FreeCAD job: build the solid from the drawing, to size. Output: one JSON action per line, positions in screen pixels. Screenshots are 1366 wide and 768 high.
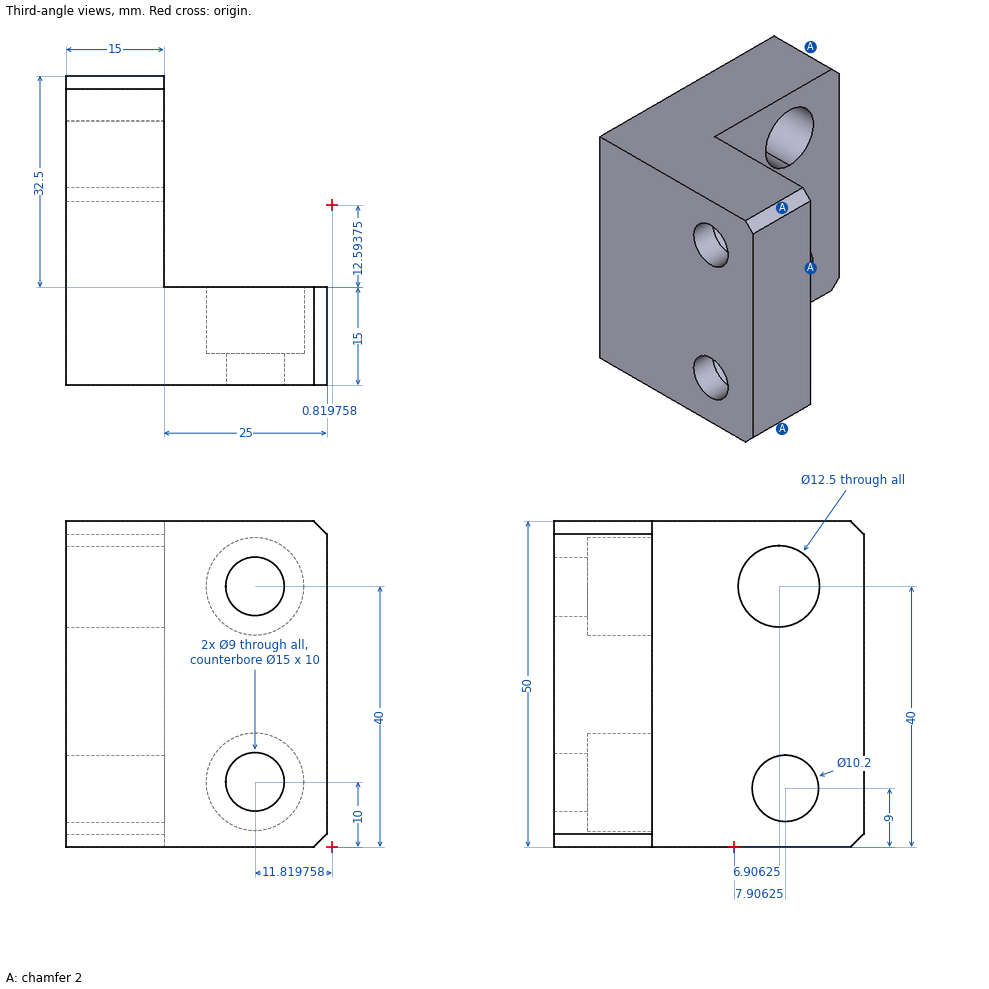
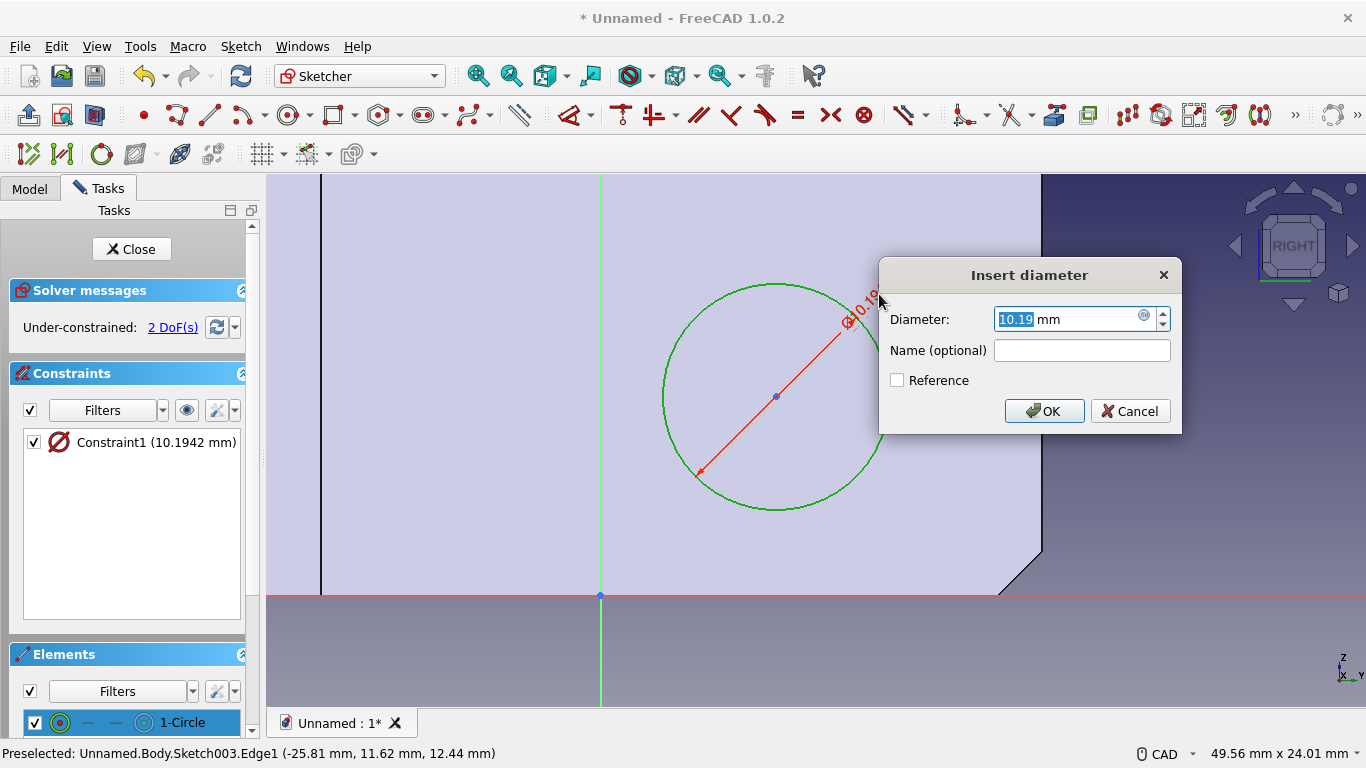
{"action": "type", "text": "10.2"}
{"action": "key", "text": "Return"}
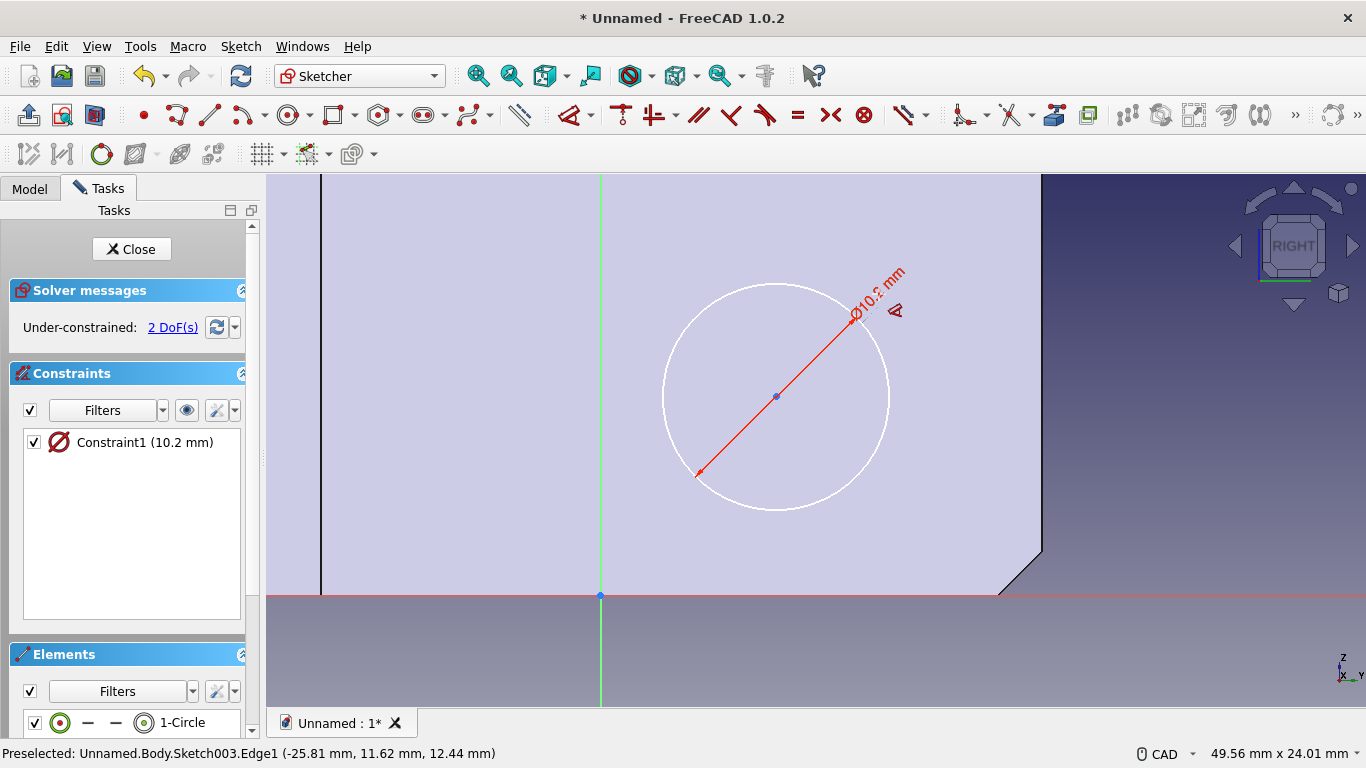
{"action": "left_click", "coordinate": [776, 397]}
{"action": "left_click", "coordinate": [567, 496]}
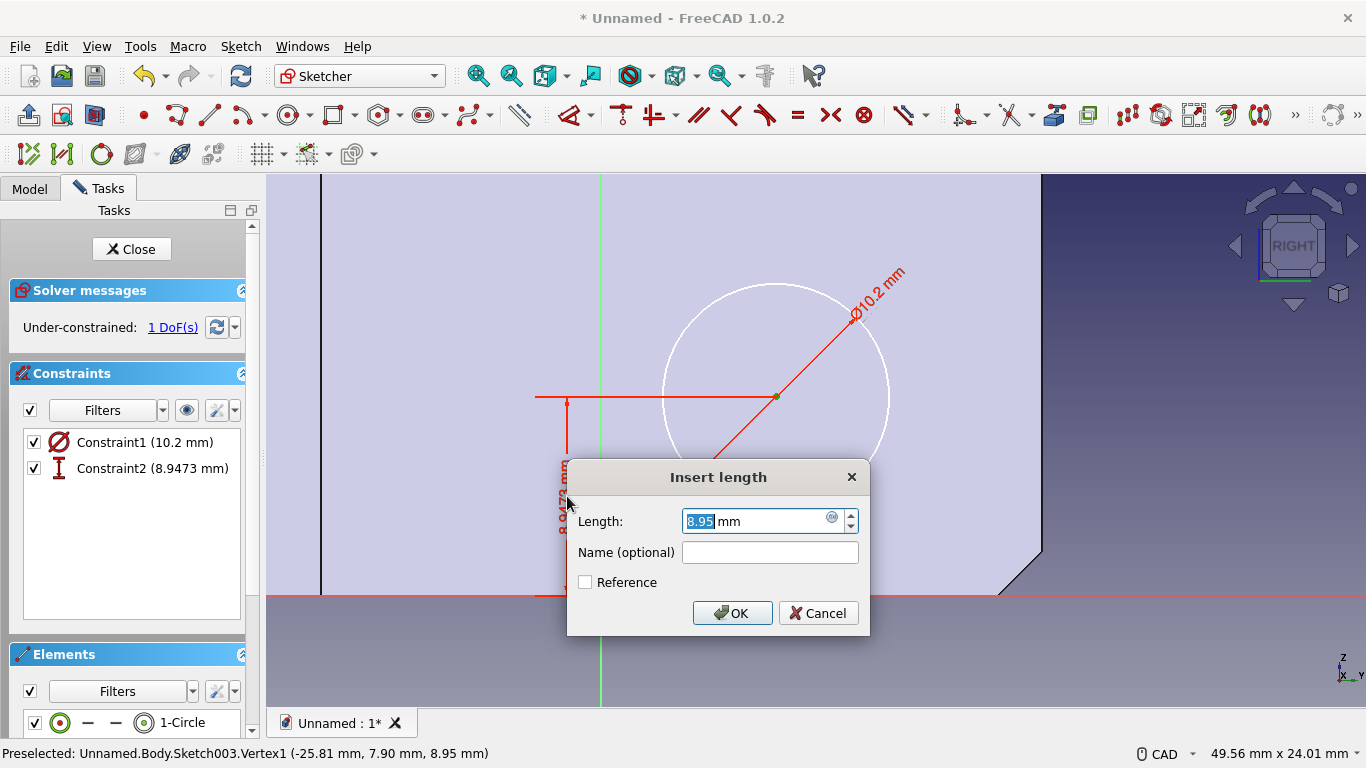
{"action": "type", "text": "9"}
{"action": "key", "text": "Return"}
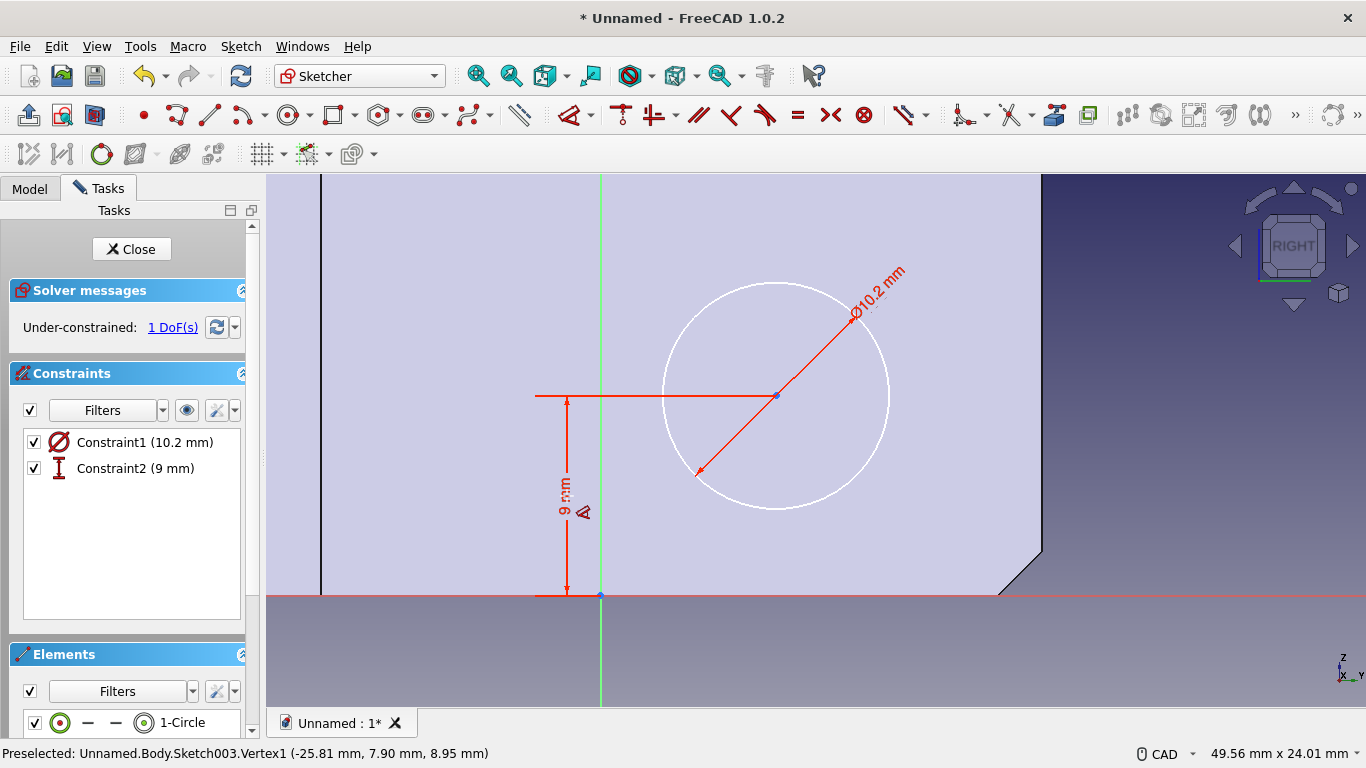
{"action": "left_click", "coordinate": [776, 396]}
{"action": "left_click", "coordinate": [688, 630]}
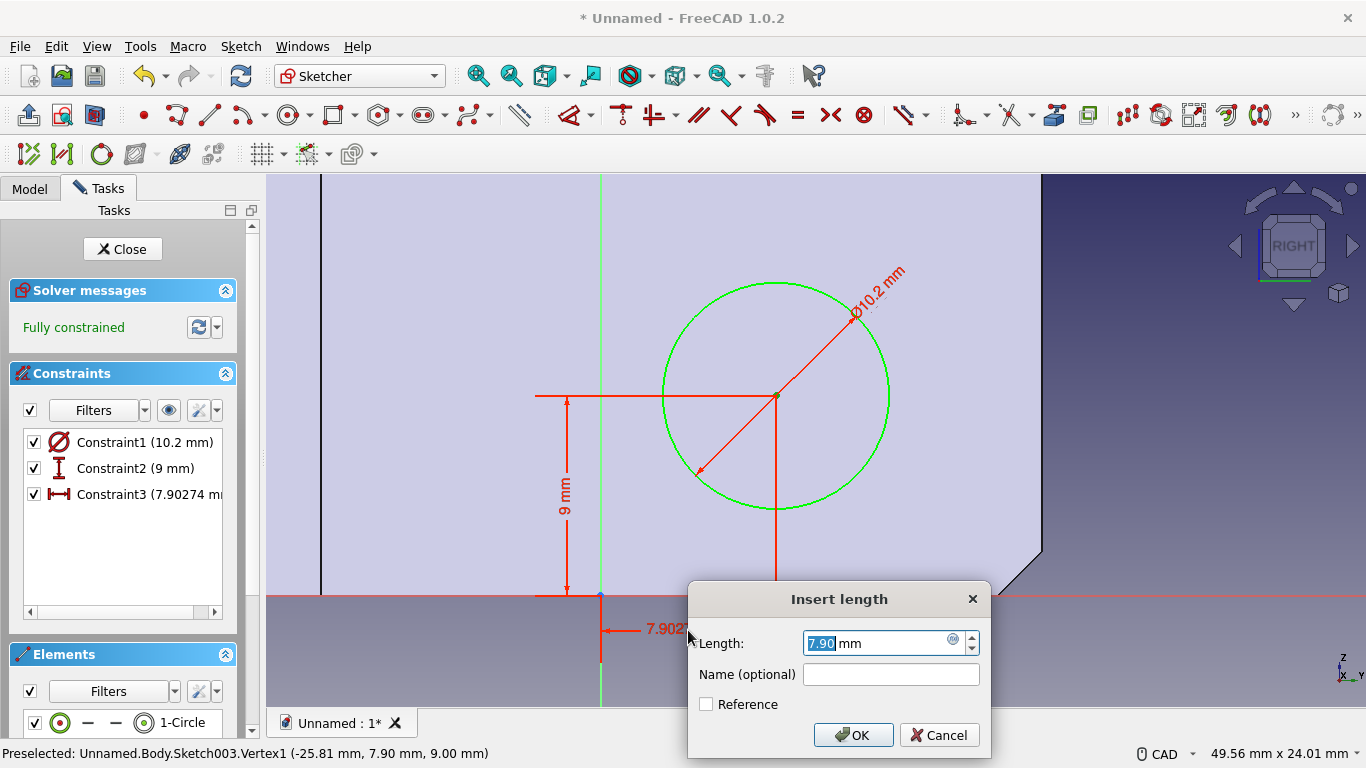
{"action": "type", "text": "7.90625"}
{"action": "key", "text": "Return"}
{"action": "key", "text": "Escape"}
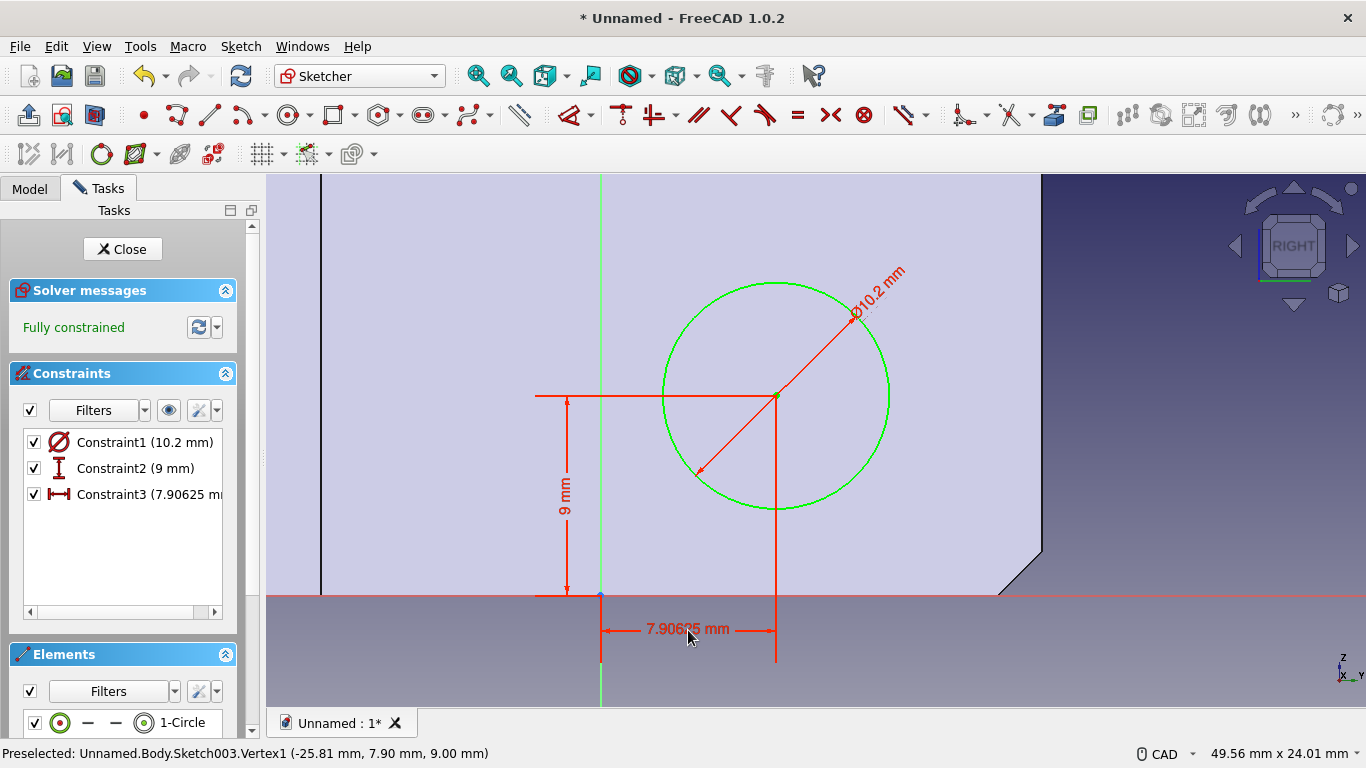
{"action": "left_click", "coordinate": [123, 249]}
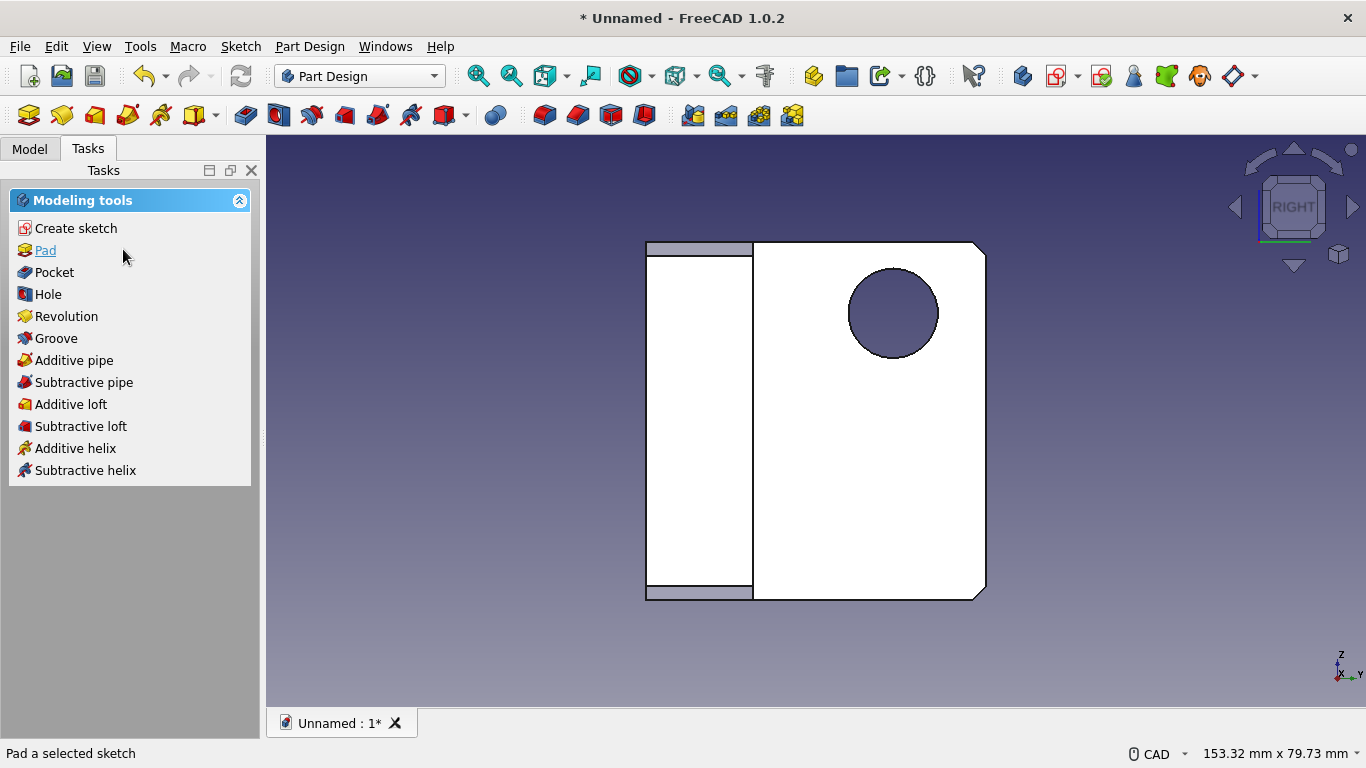
{"action": "left_click", "coordinate": [246, 116]}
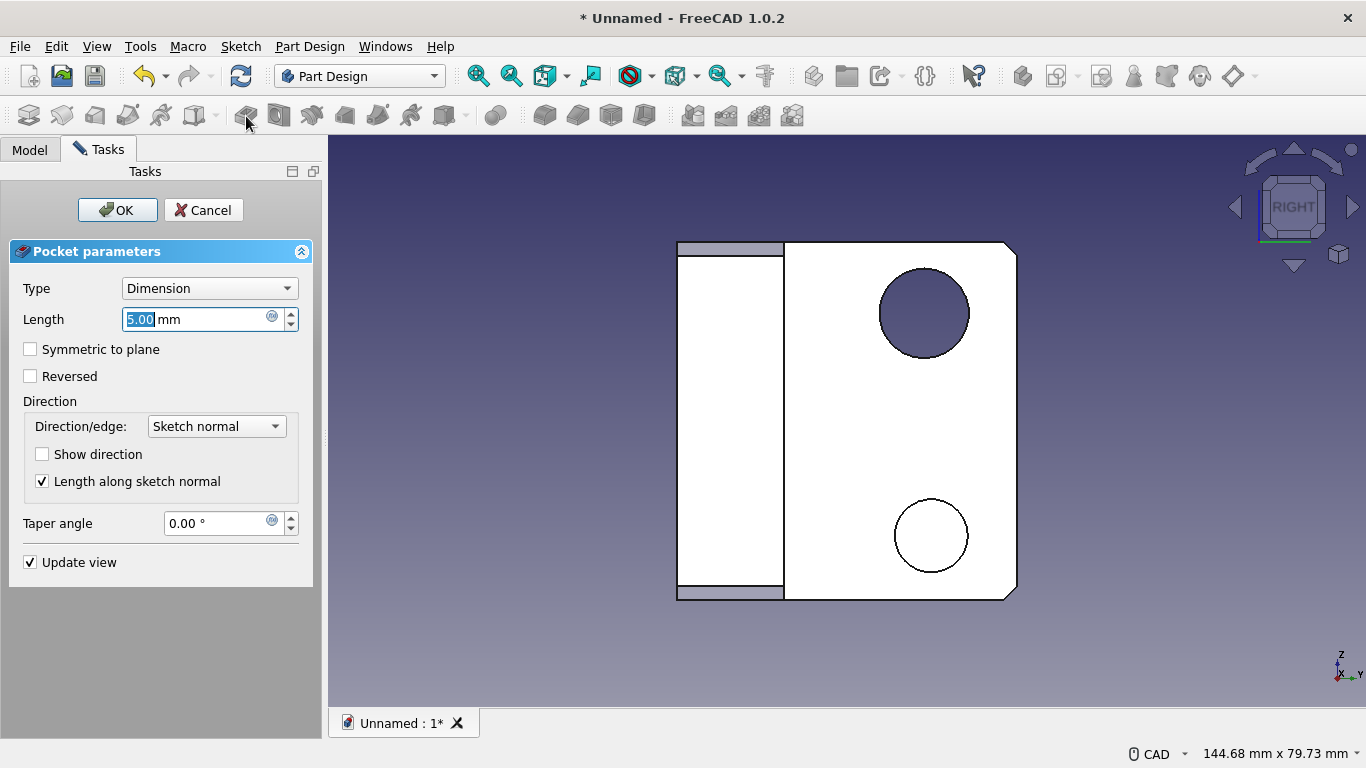
{"action": "left_click", "coordinate": [210, 288]}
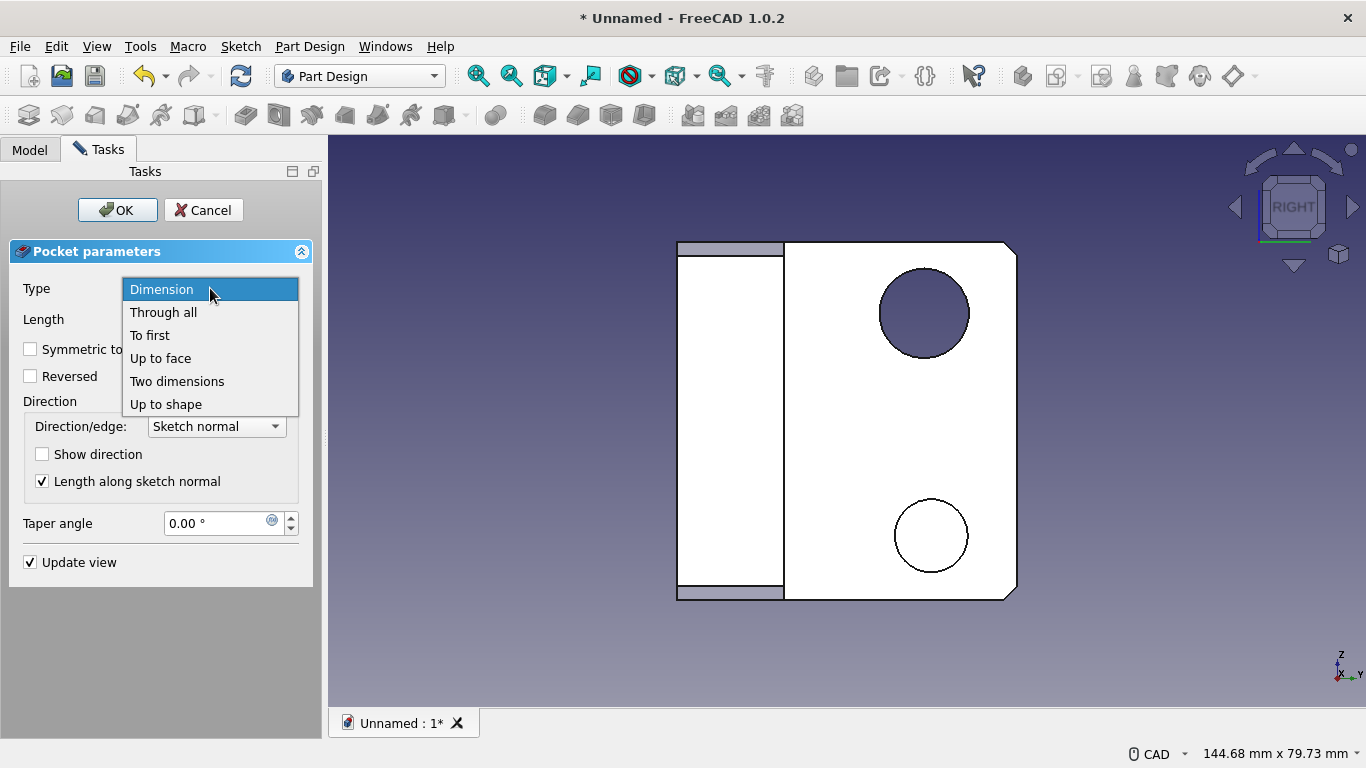
{"action": "left_click", "coordinate": [208, 312]}